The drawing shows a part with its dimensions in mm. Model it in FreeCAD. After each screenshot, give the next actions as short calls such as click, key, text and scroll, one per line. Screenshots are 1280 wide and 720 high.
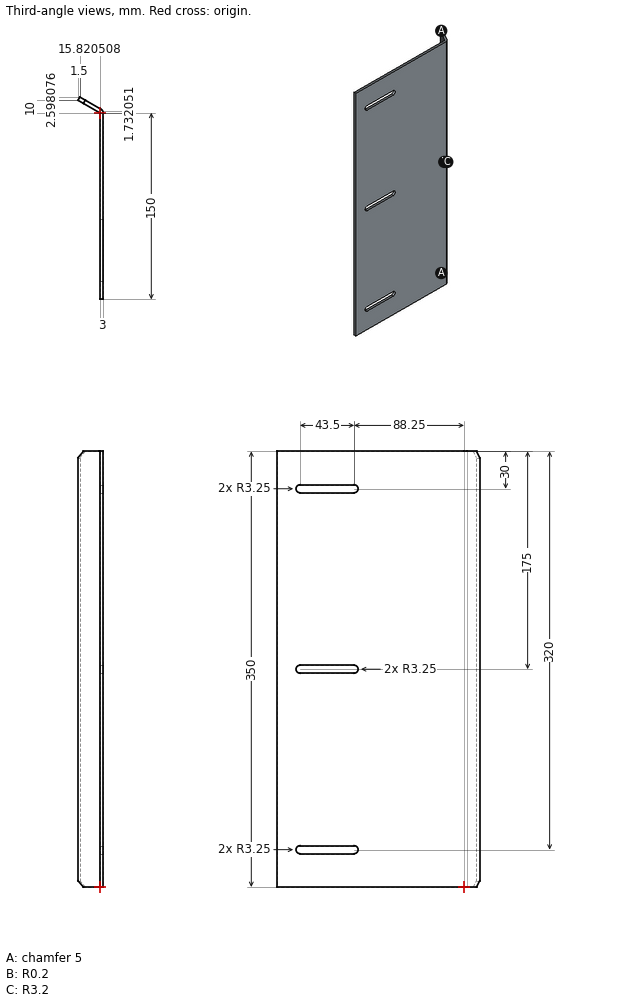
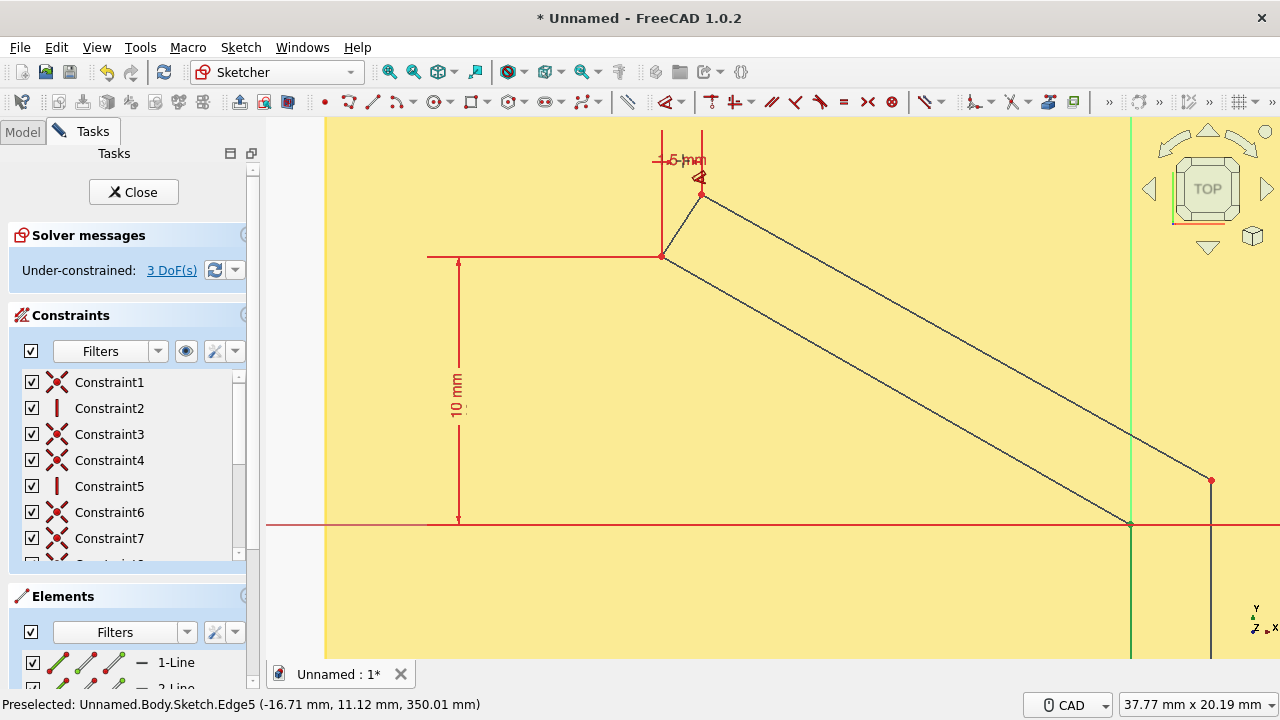
scroll(686, 229, down, 13)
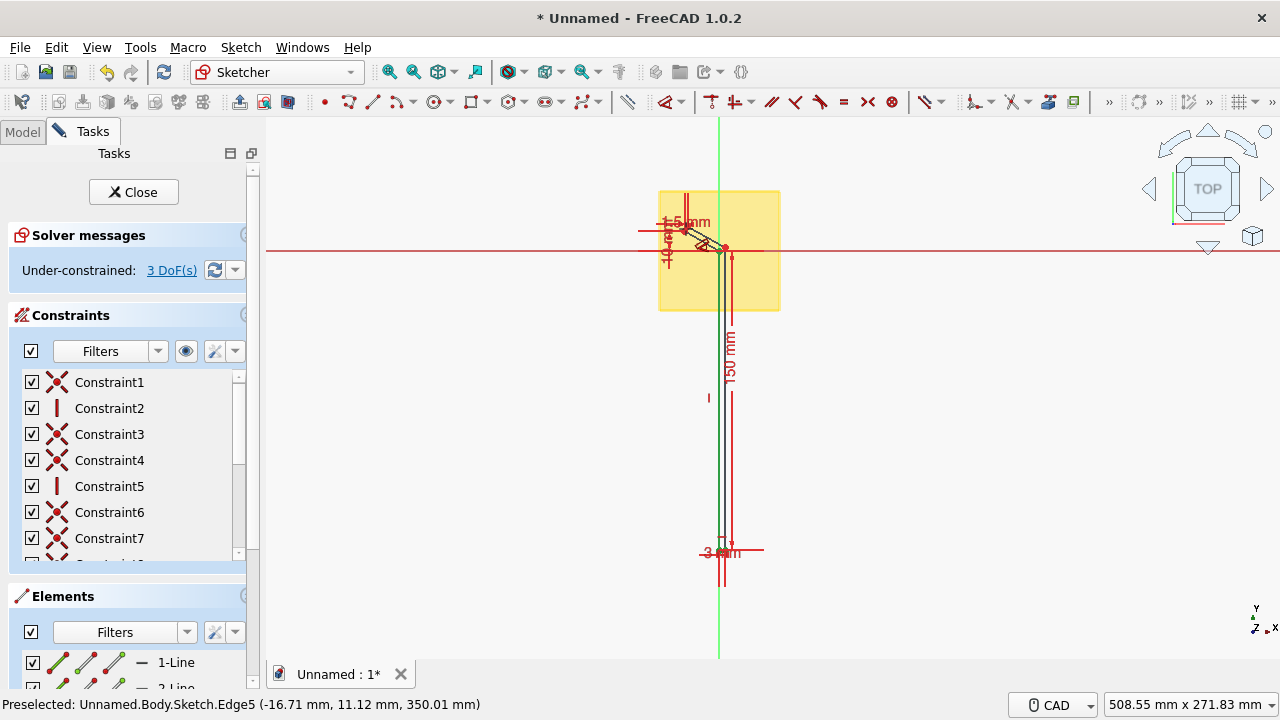
scroll(725, 248, up, 13)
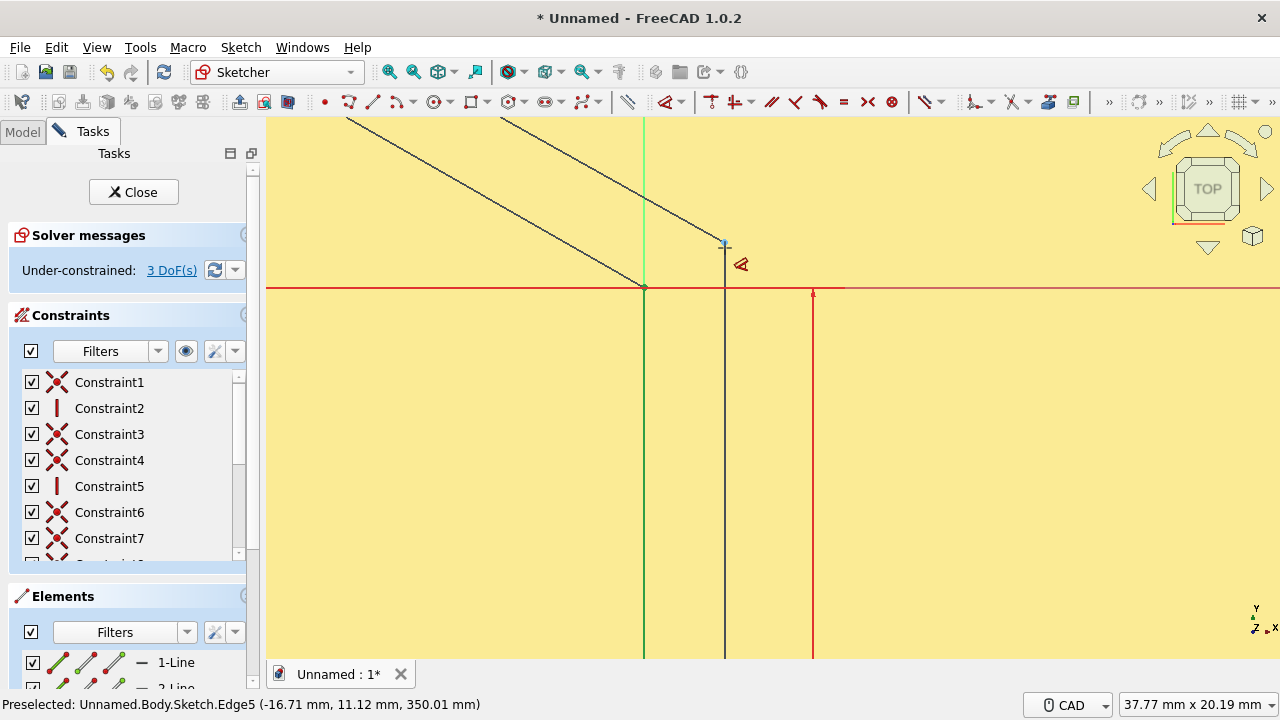
click(725, 243)
click(759, 265)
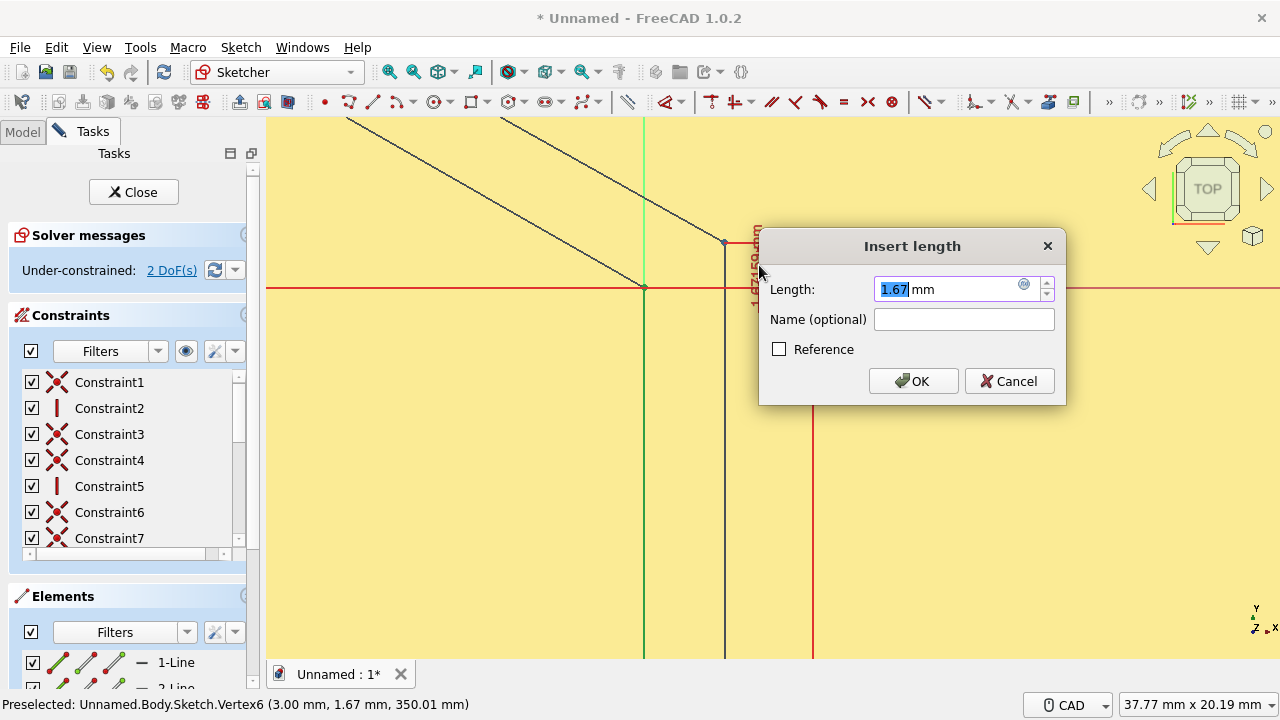
text(1.732051)
key(Return)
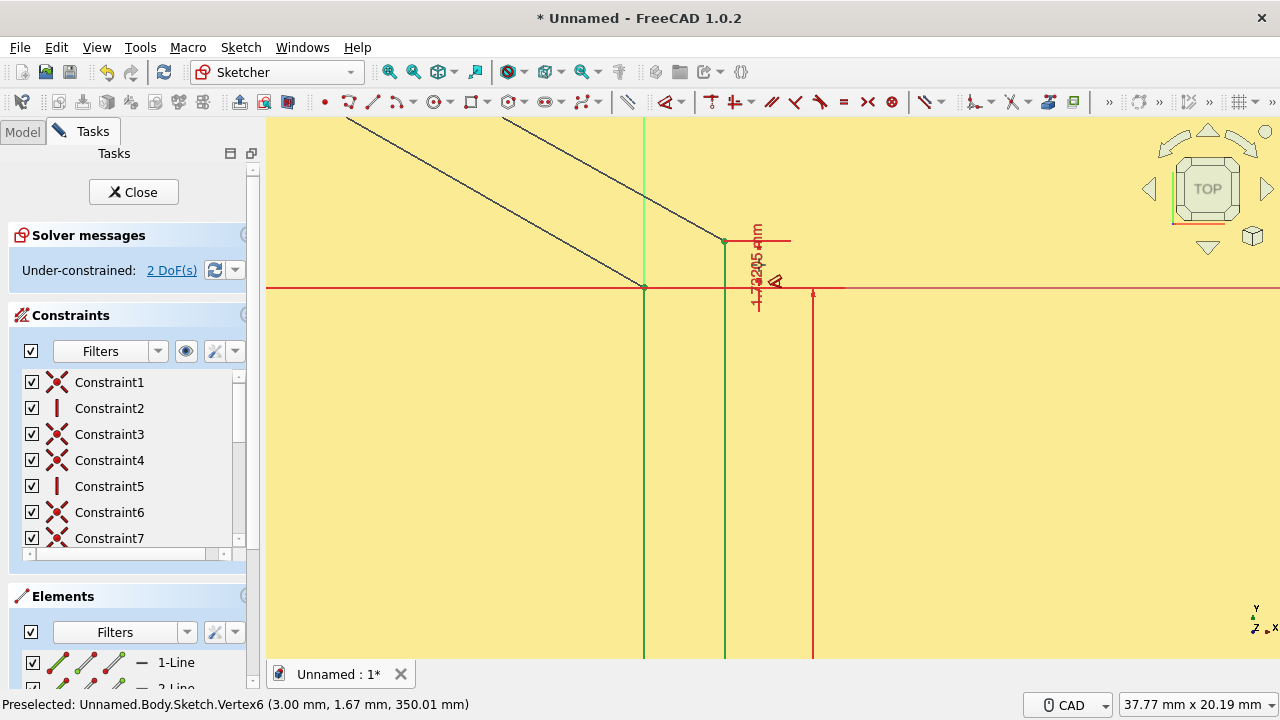
scroll(725, 248, down, 13)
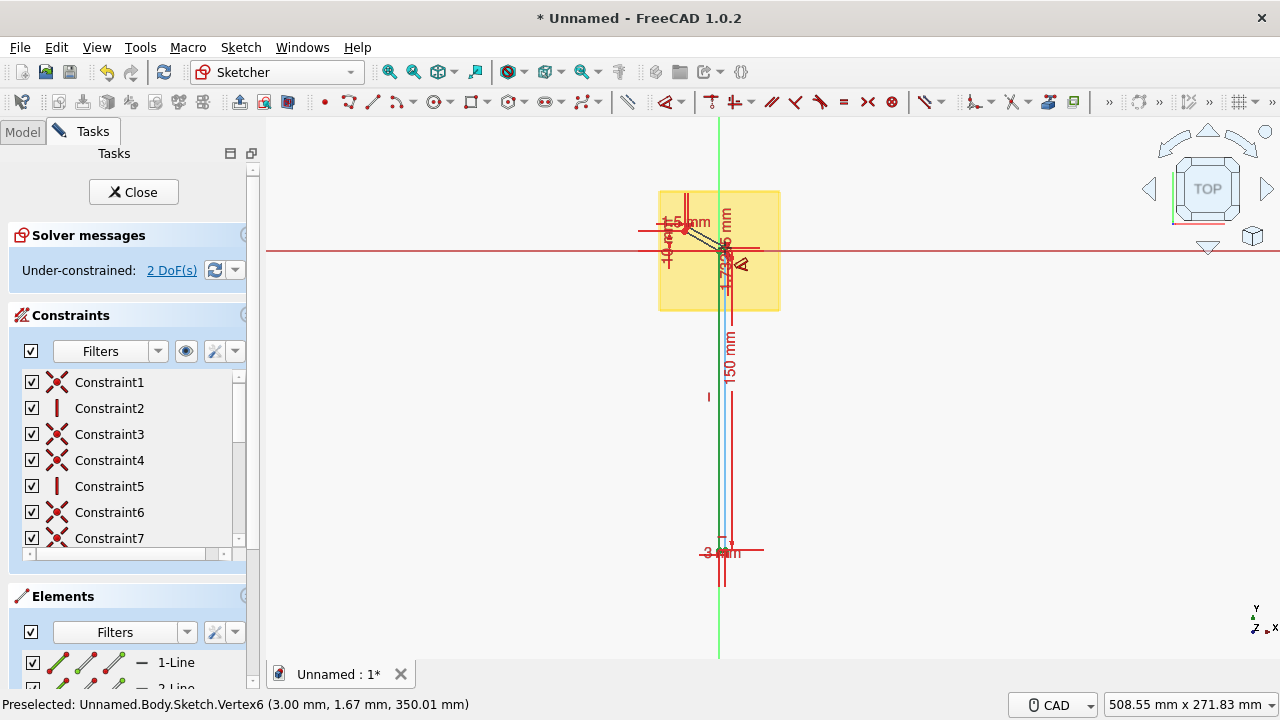
scroll(687, 228, up, 11)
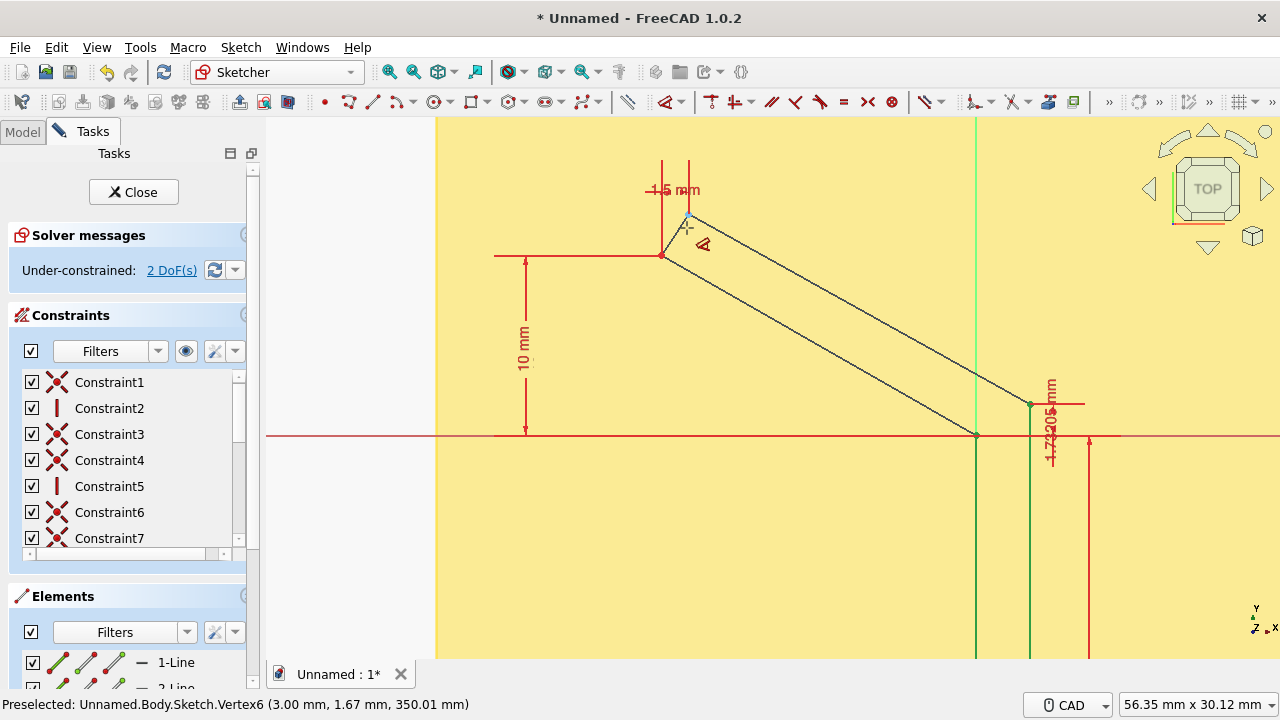
click(681, 227)
click(628, 235)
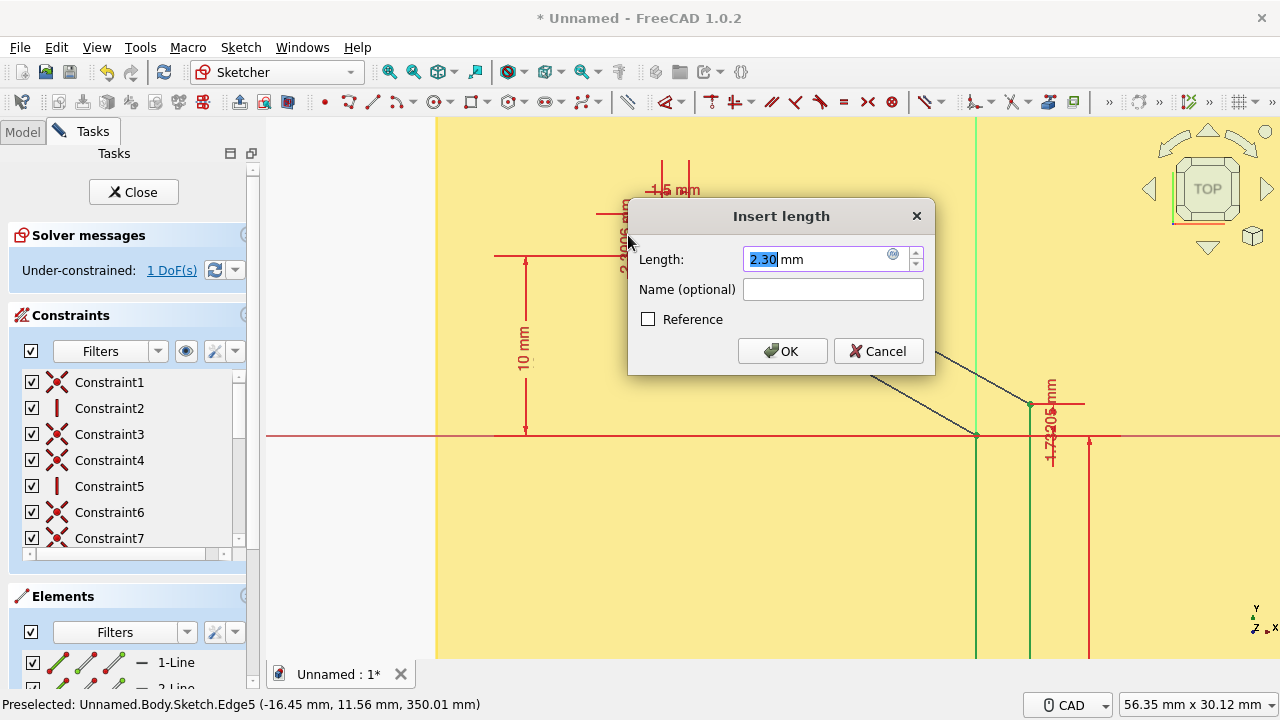
text(2.598076)
key(Return)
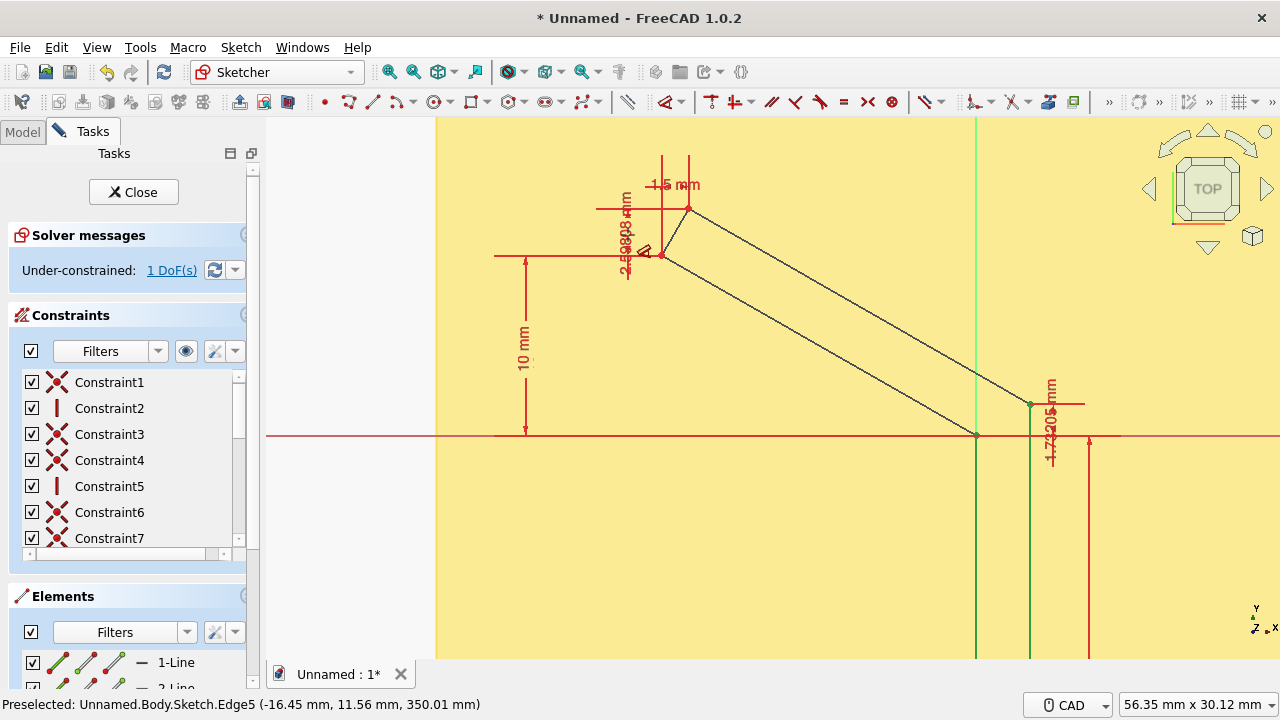
scroll(687, 228, down, 11)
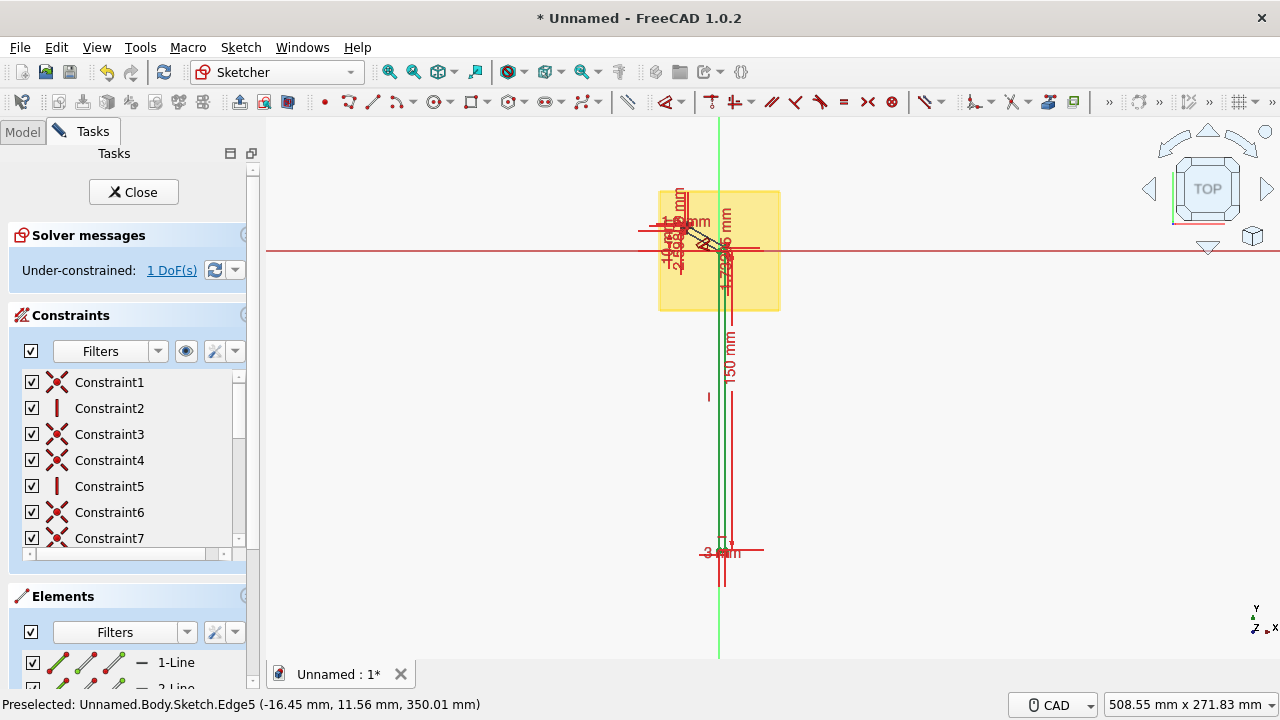
scroll(688, 226, up, 4)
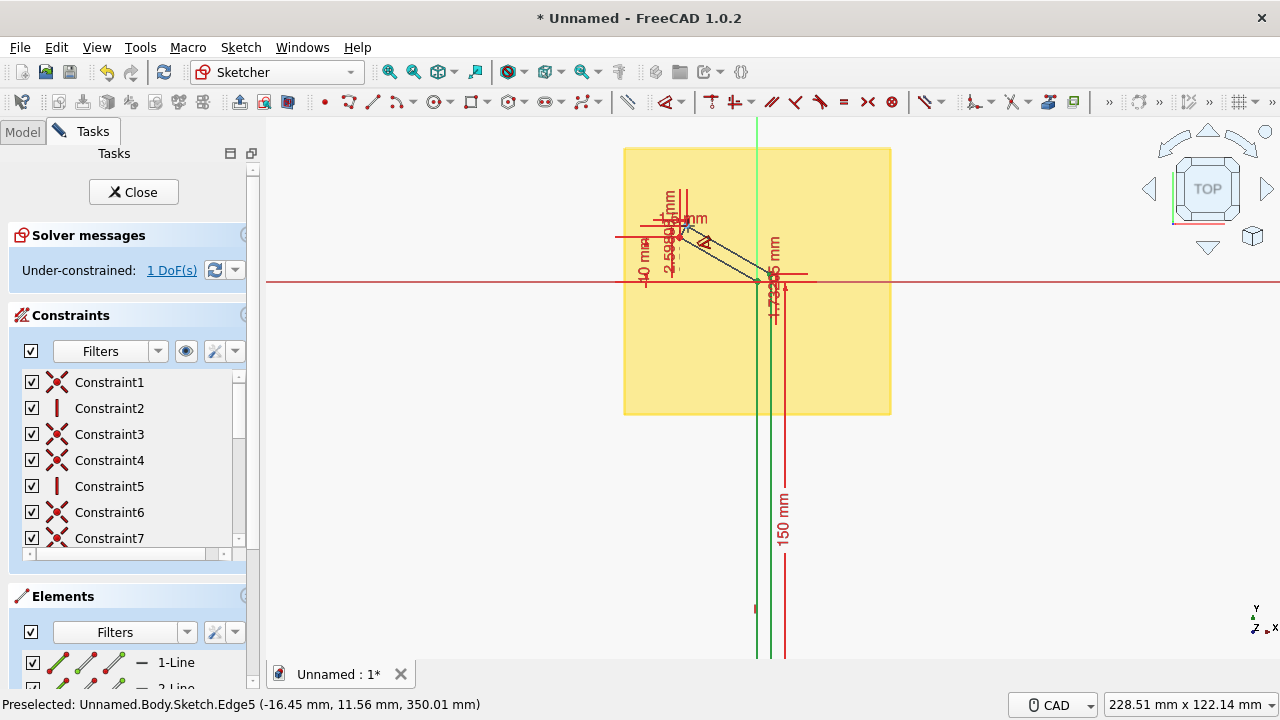
click(687, 226)
click(722, 192)